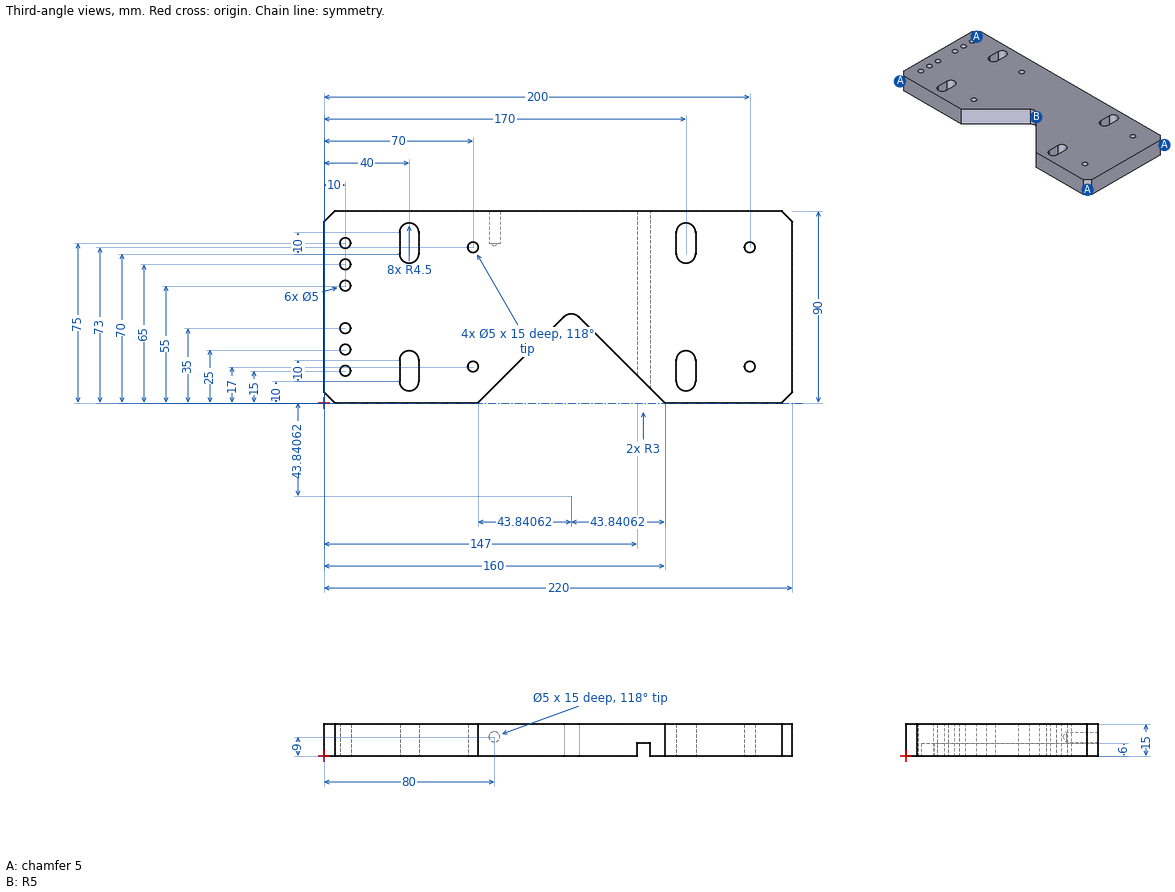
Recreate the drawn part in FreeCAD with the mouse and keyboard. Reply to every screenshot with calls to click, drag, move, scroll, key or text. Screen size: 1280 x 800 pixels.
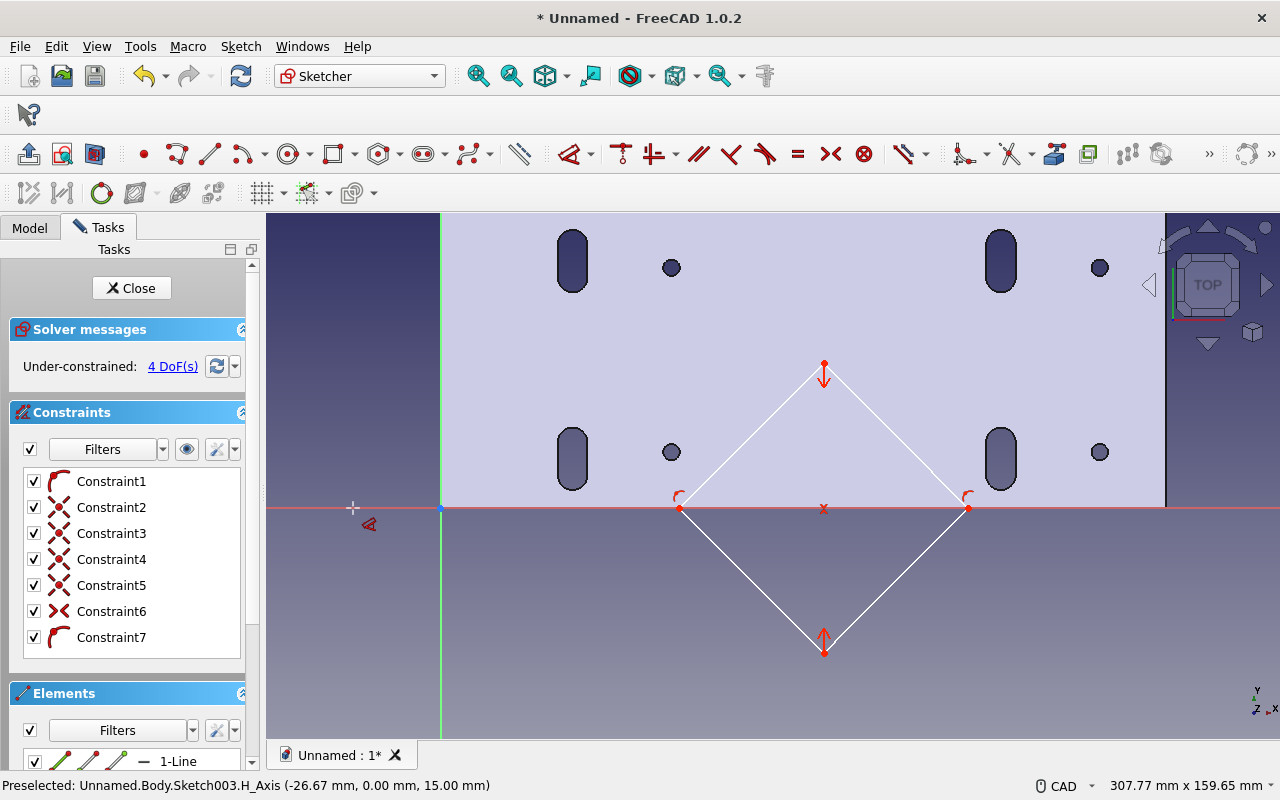
click(968, 508)
click(583, 542)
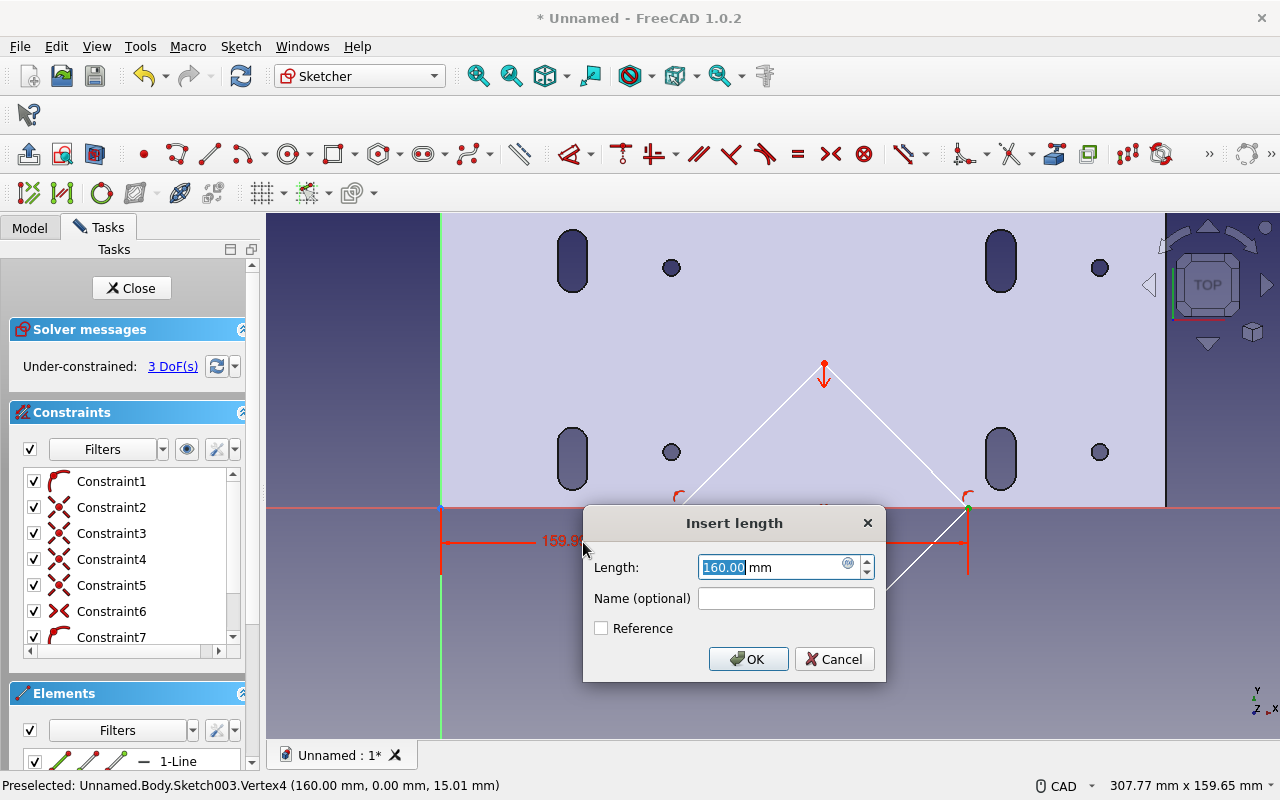
text(160)
key(Return)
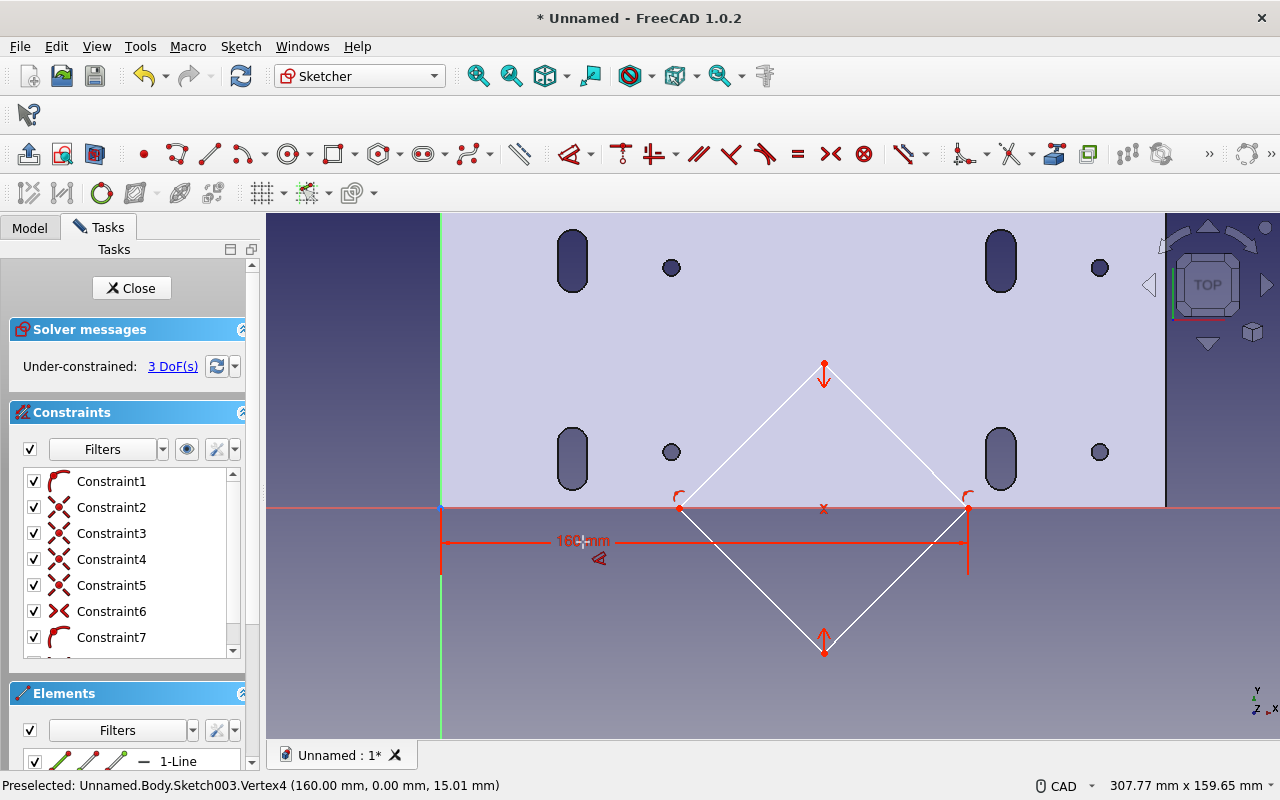
click(824, 653)
click(407, 581)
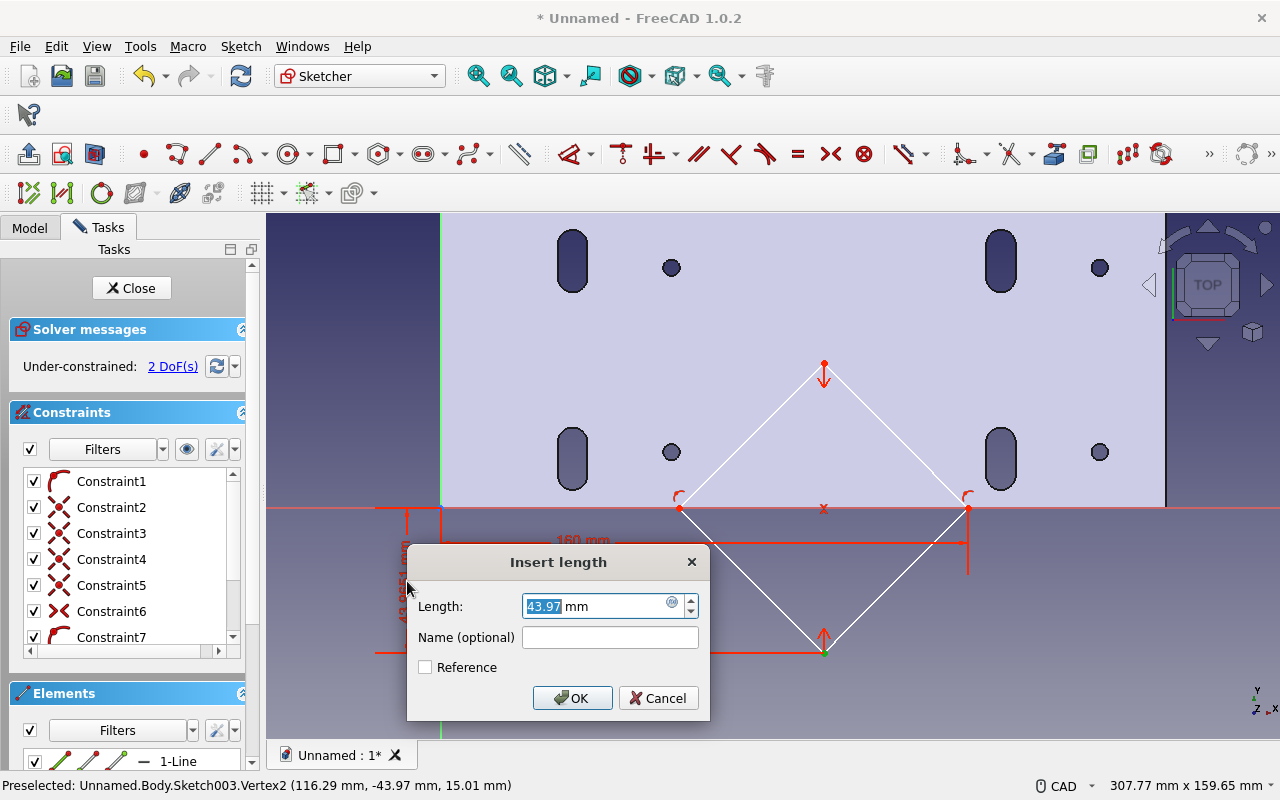
text(43.84062)
key(Return)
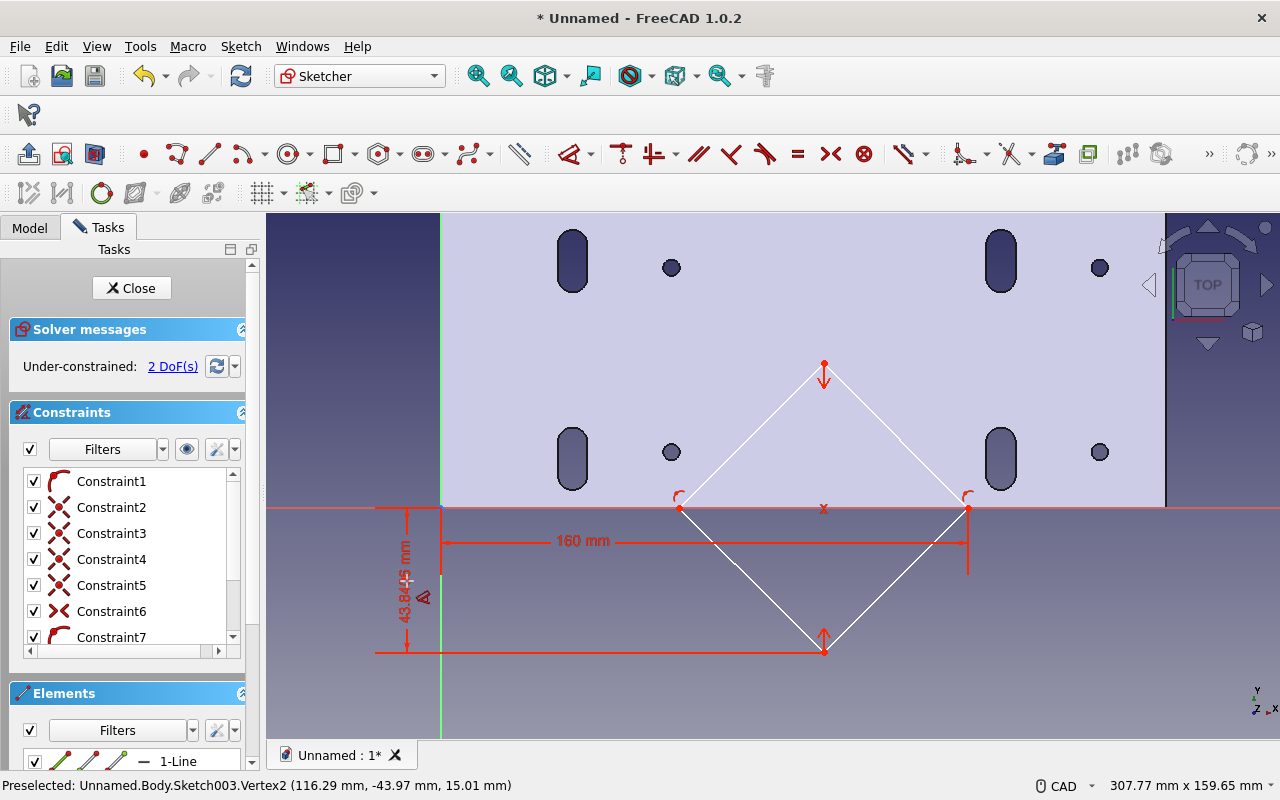
click(722, 552)
click(751, 687)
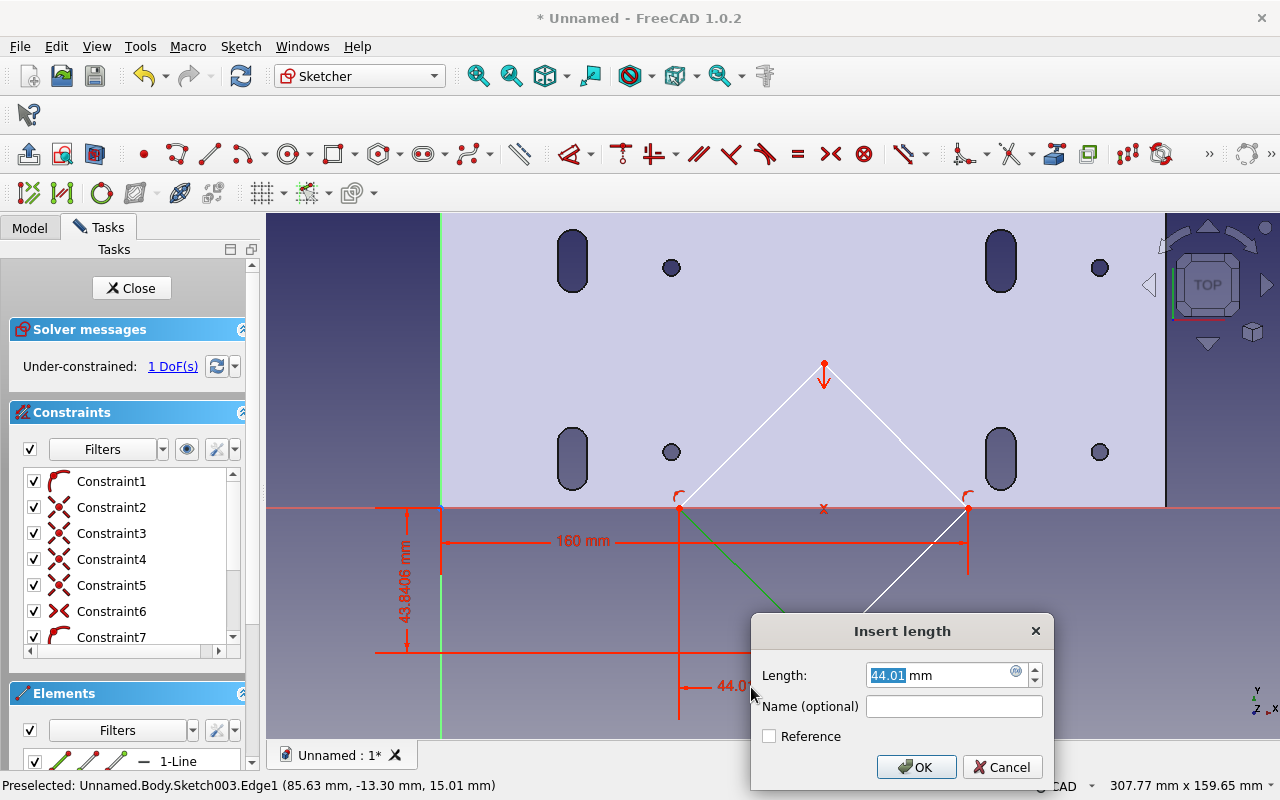
text(43.84062)
key(Return)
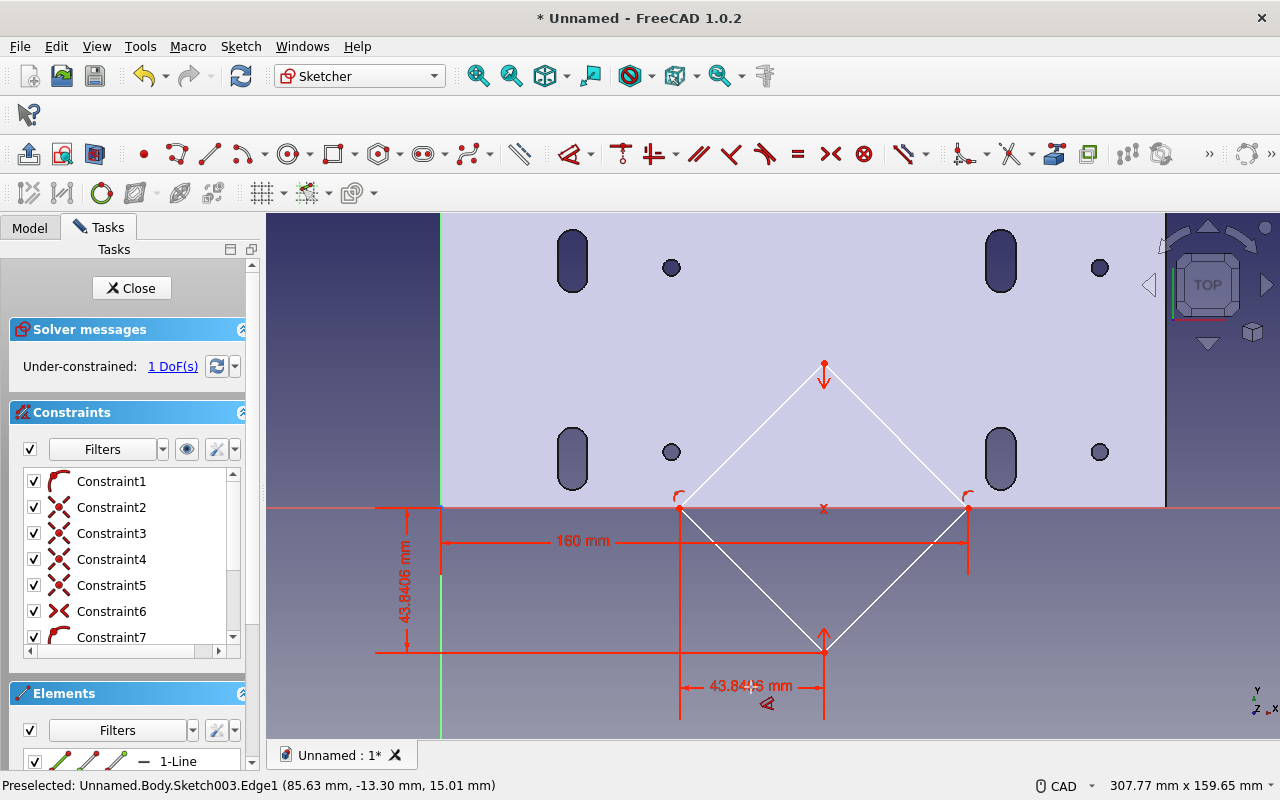
click(867, 609)
click(896, 687)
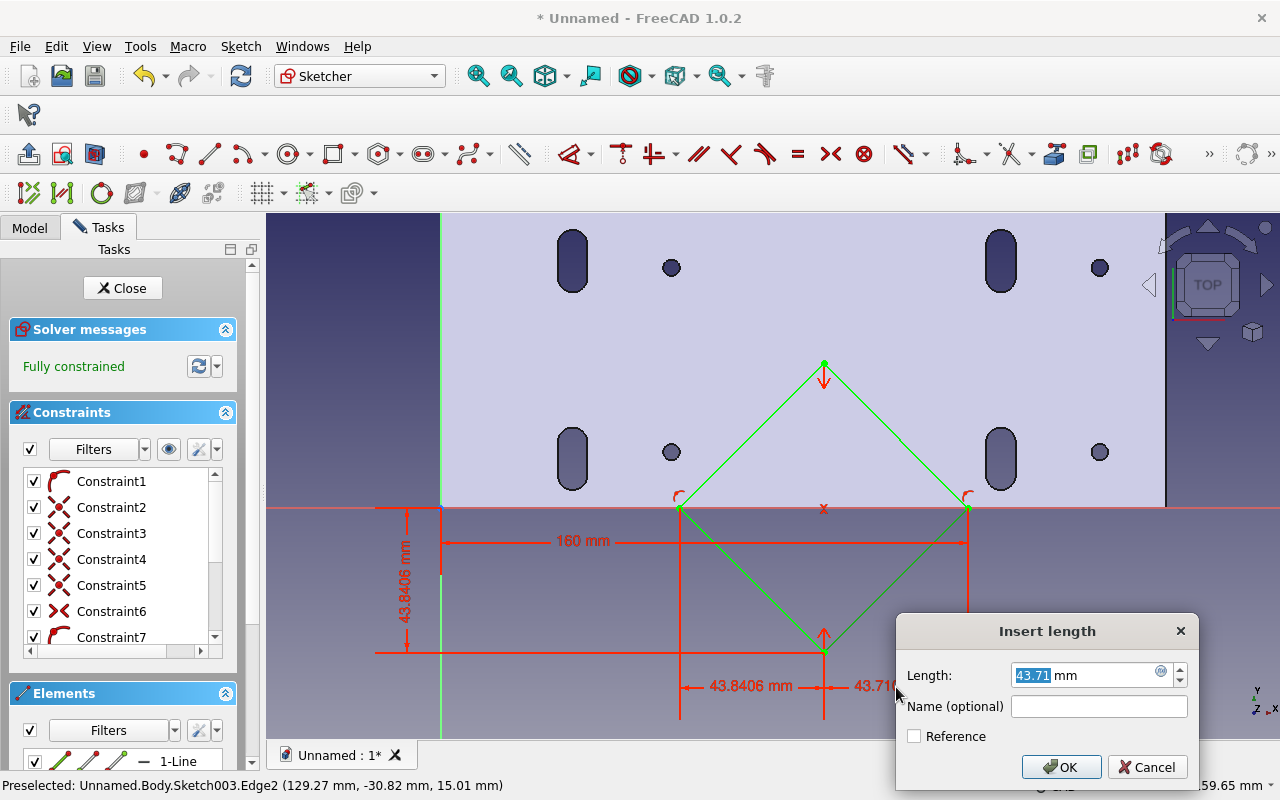
text(43.84062)
key(Return)
key(Escape)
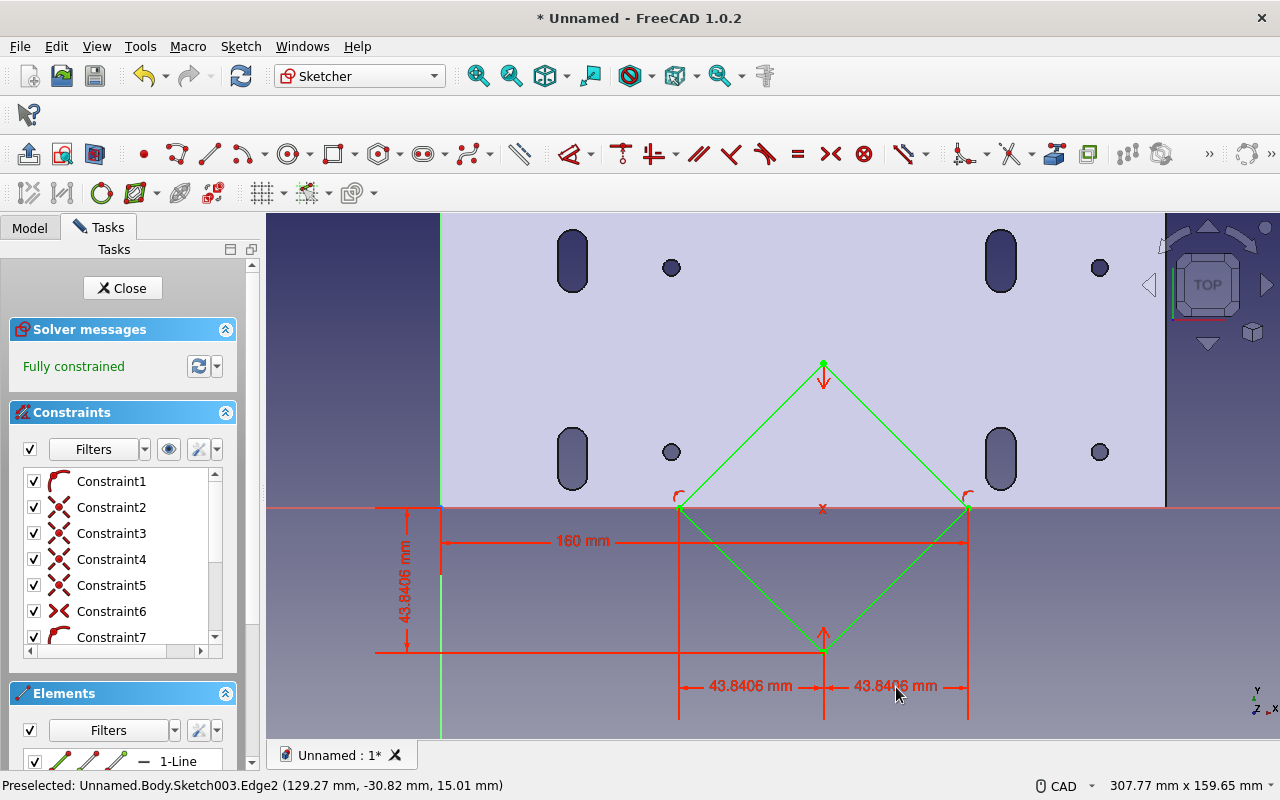
click(123, 288)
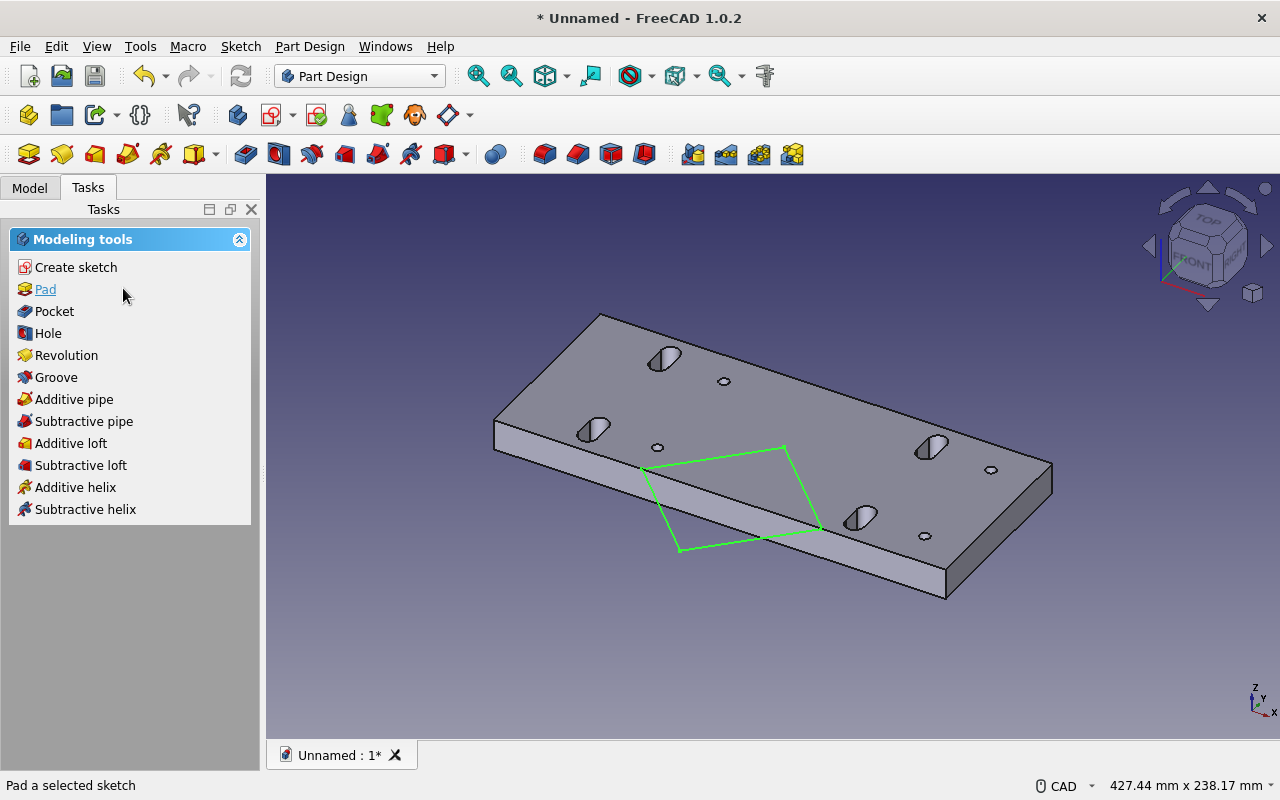
click(246, 154)